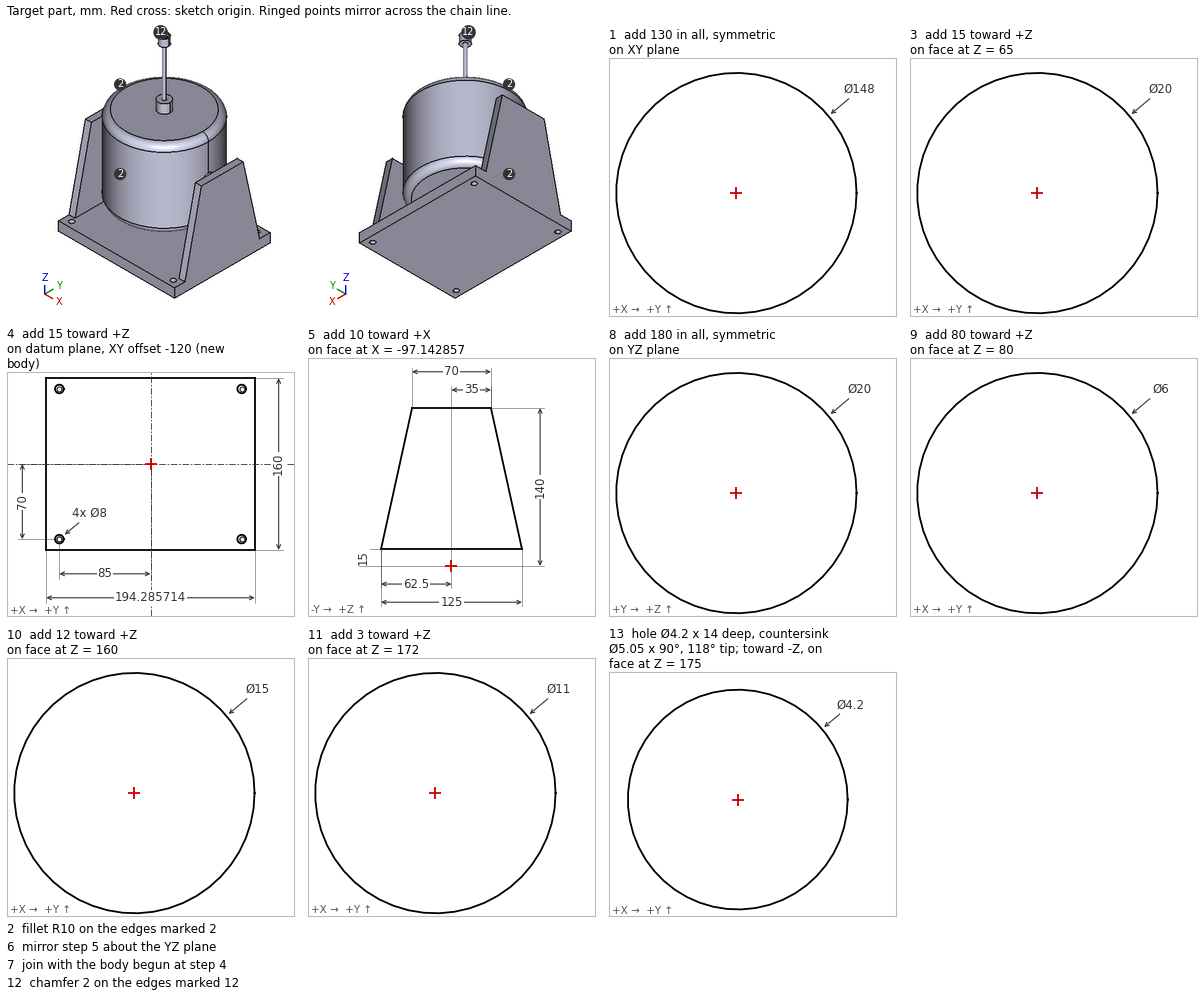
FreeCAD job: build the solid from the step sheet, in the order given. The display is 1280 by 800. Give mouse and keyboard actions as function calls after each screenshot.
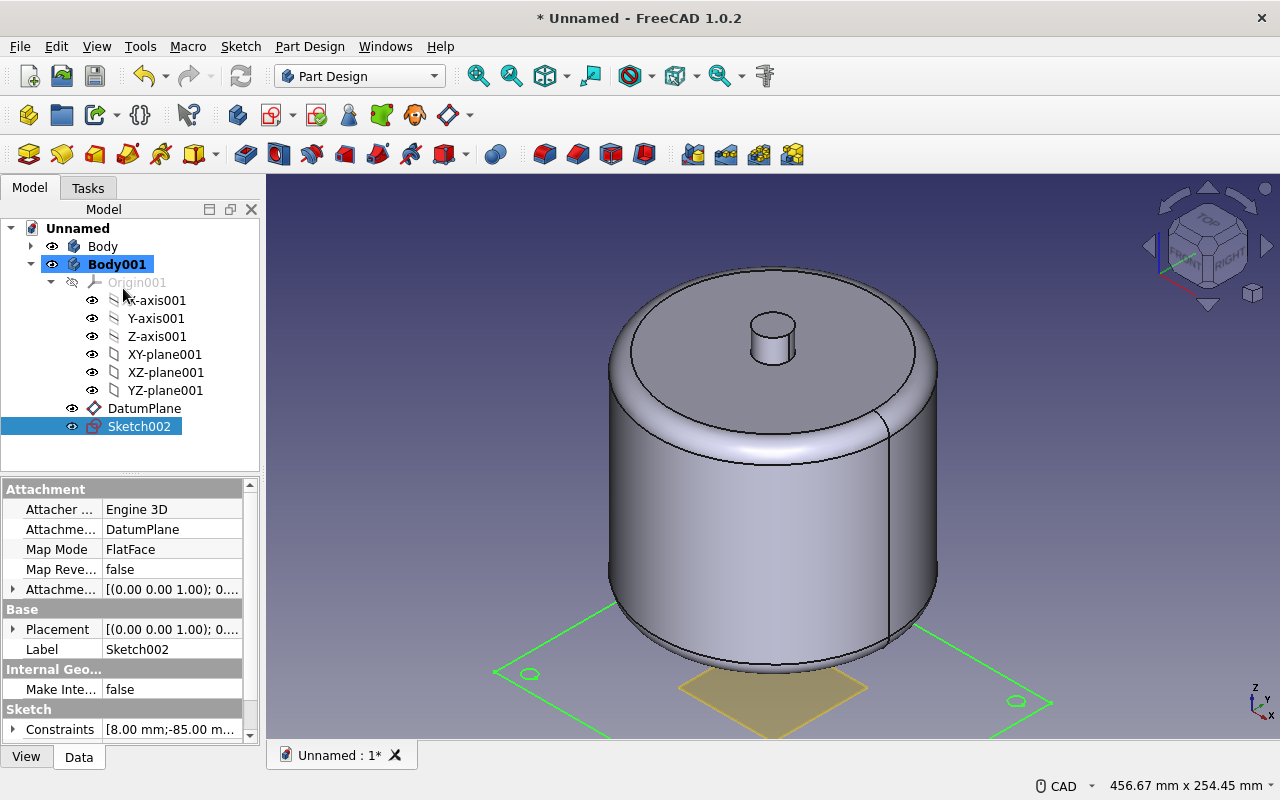
click(29, 154)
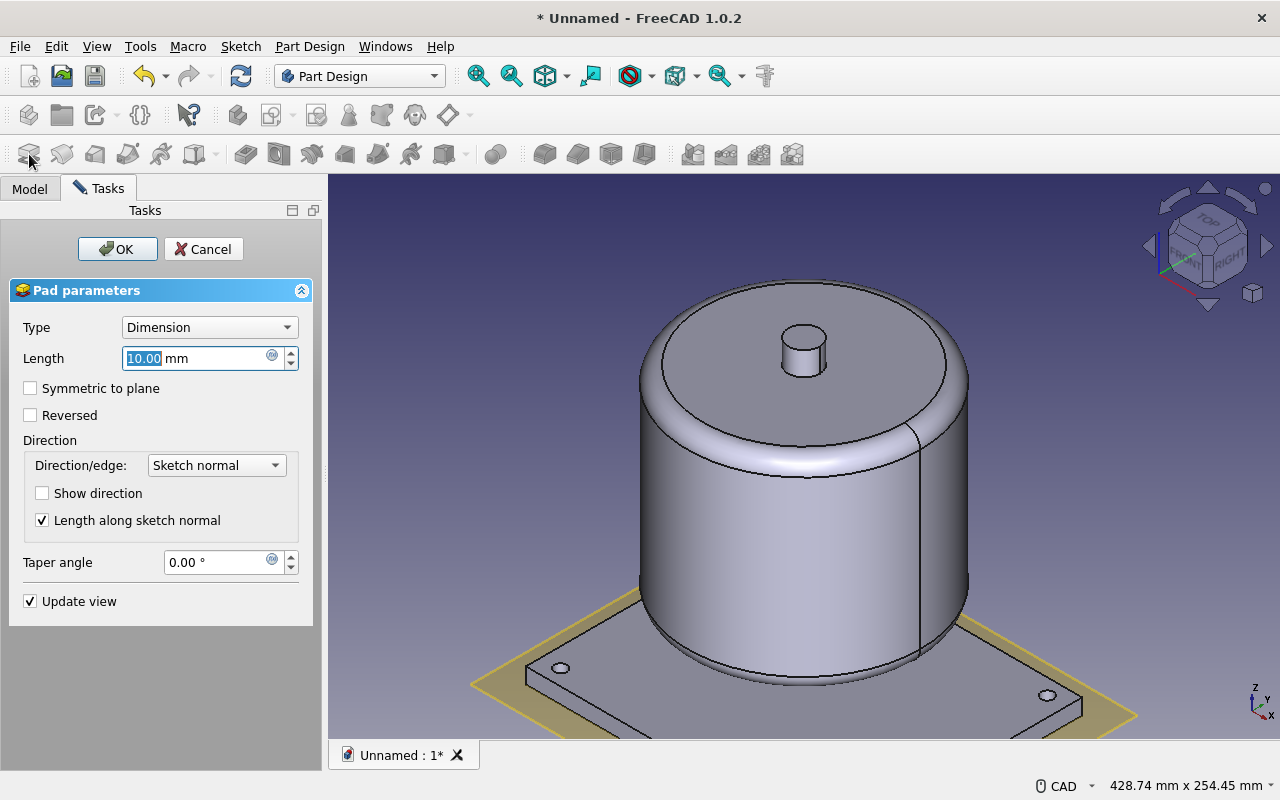
text(15)
key(Tab)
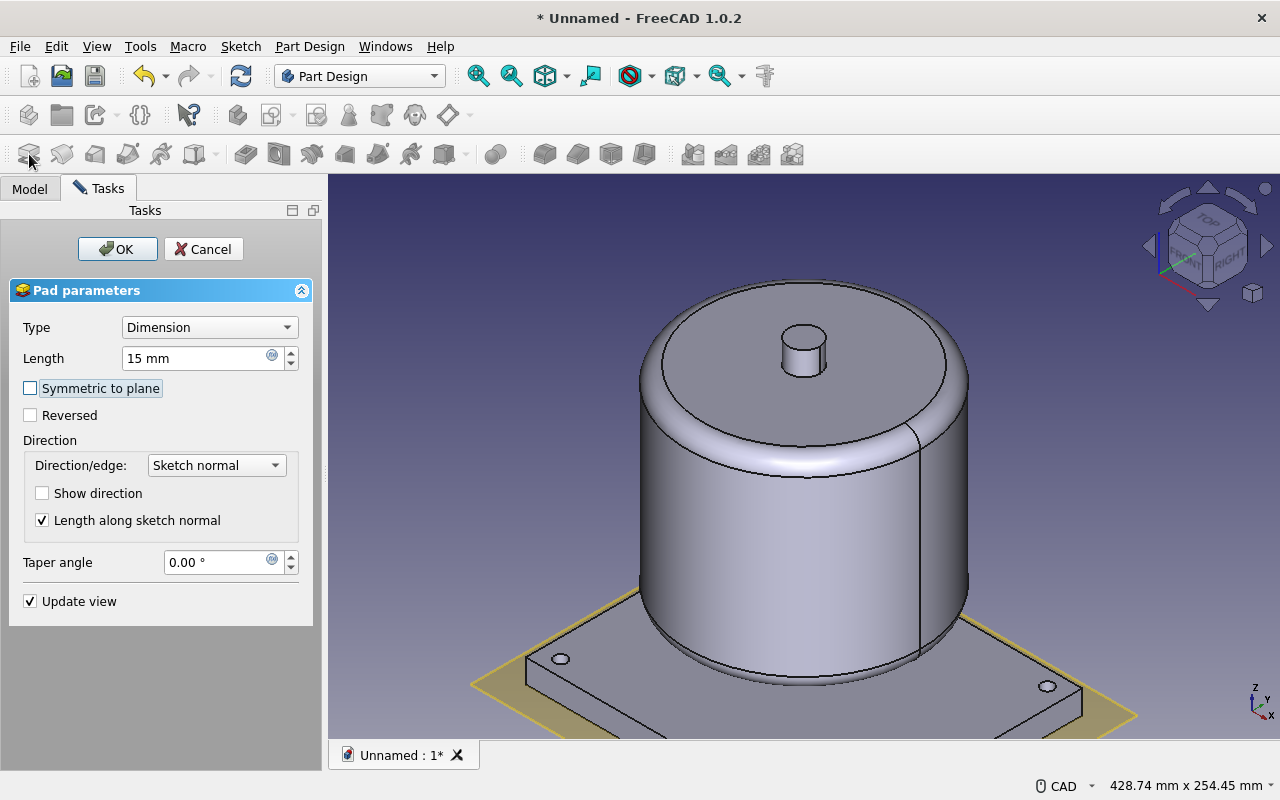
click(118, 249)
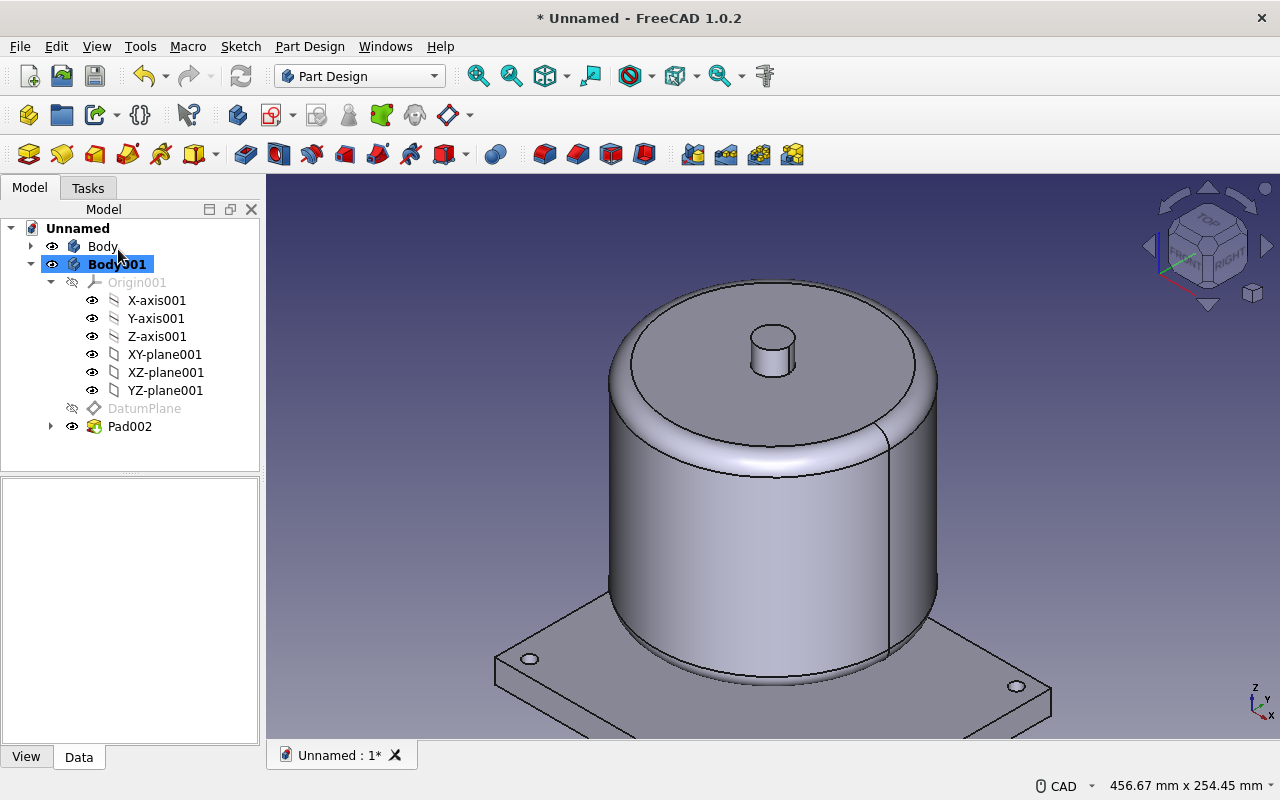
key(v)
key(f)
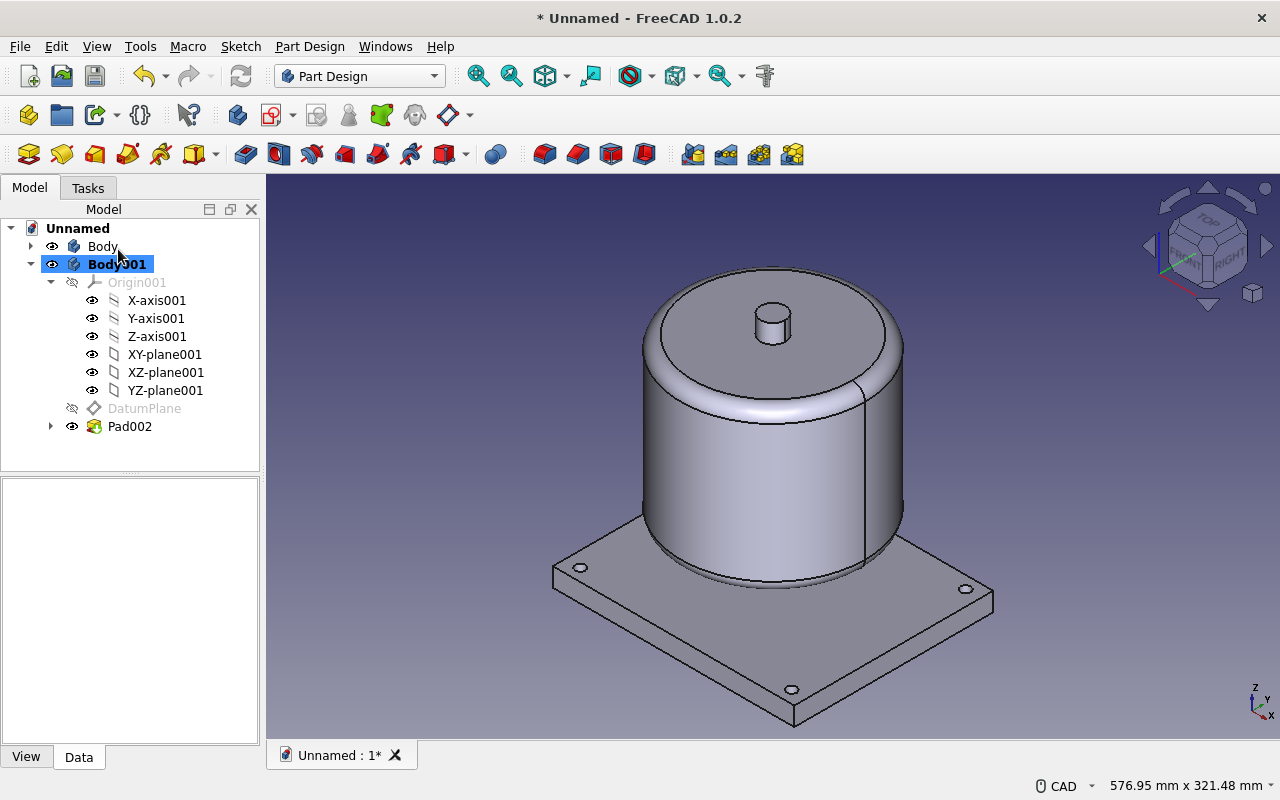
key(6)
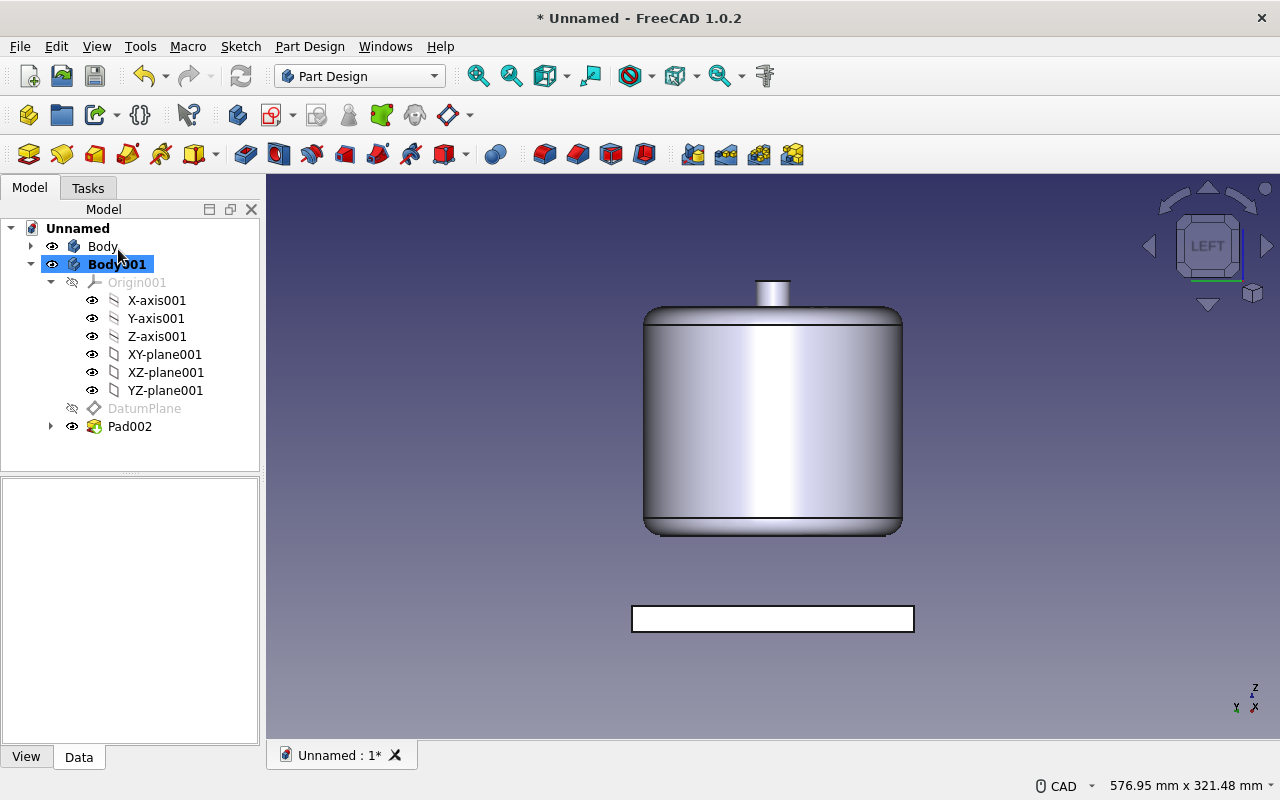
key(v)
key(f)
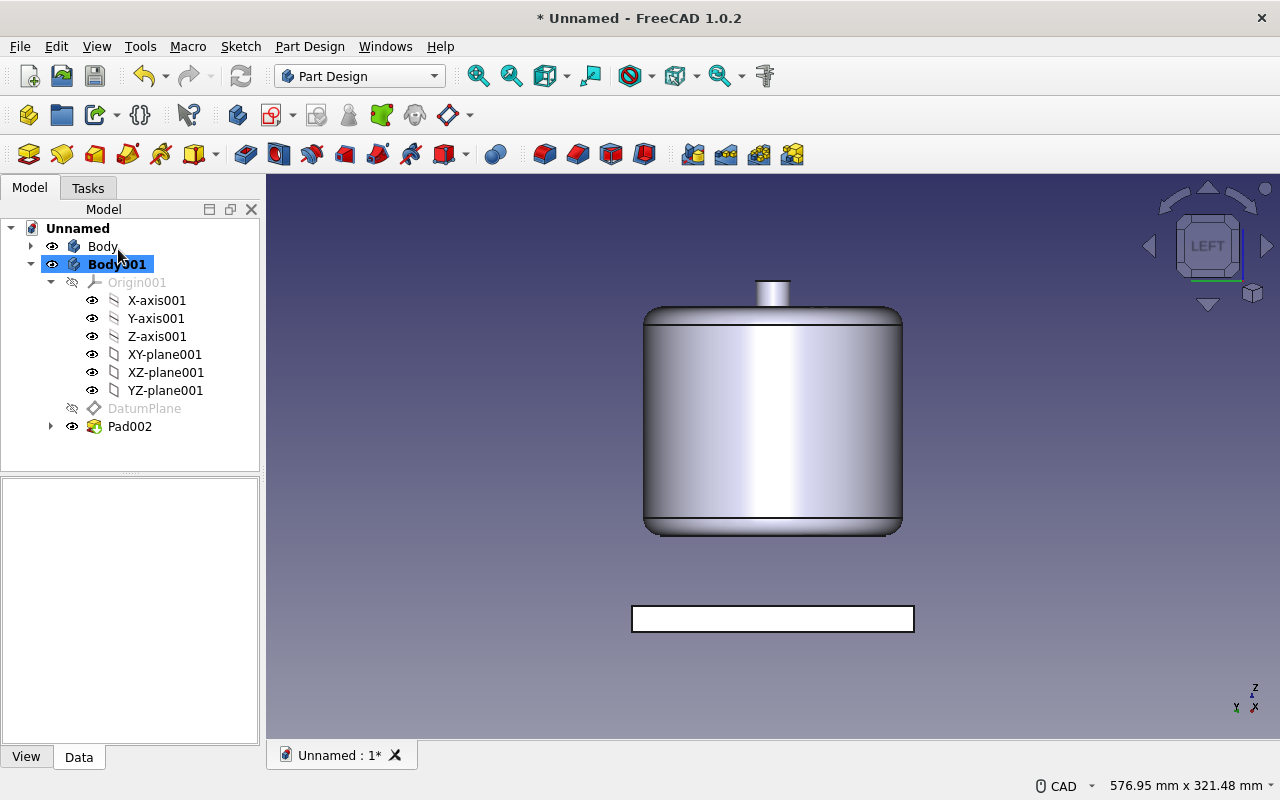
click(652, 618)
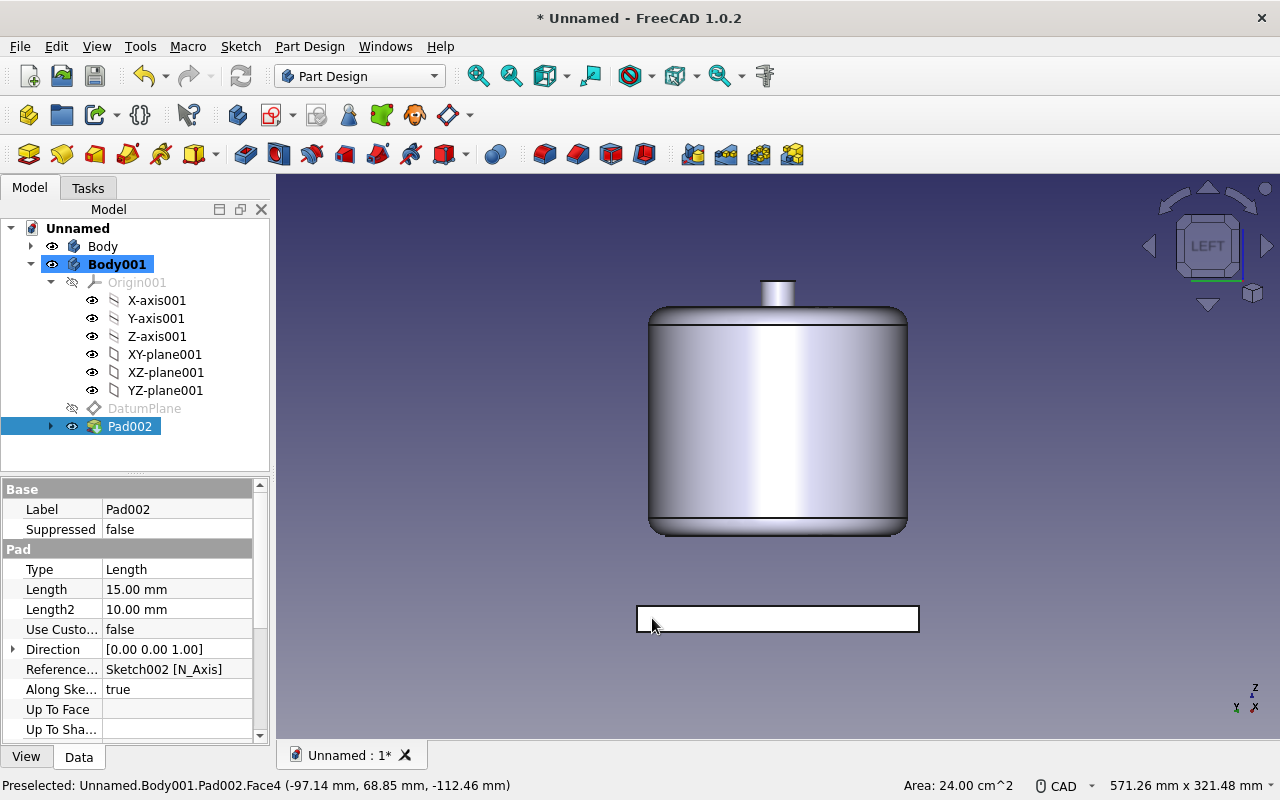
click(270, 116)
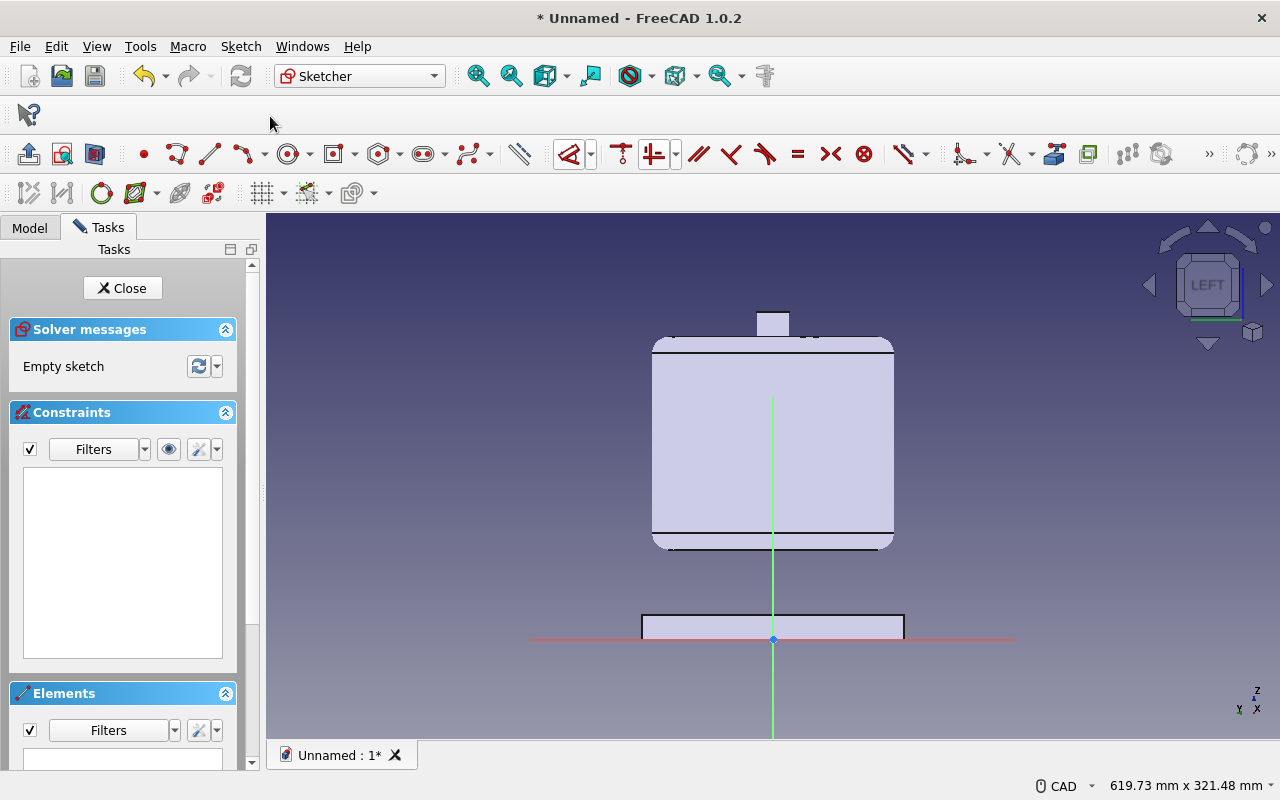
scroll(912, 625, up, 2)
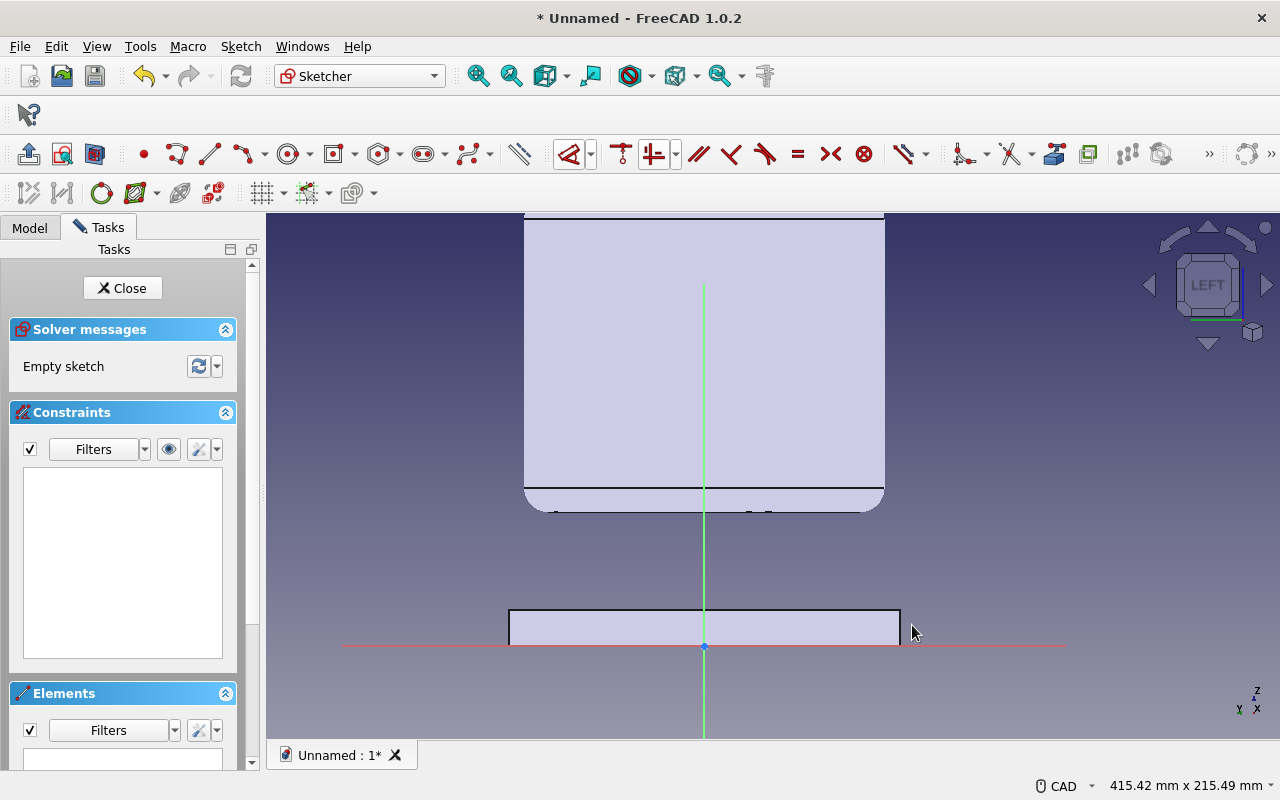
click(177, 154)